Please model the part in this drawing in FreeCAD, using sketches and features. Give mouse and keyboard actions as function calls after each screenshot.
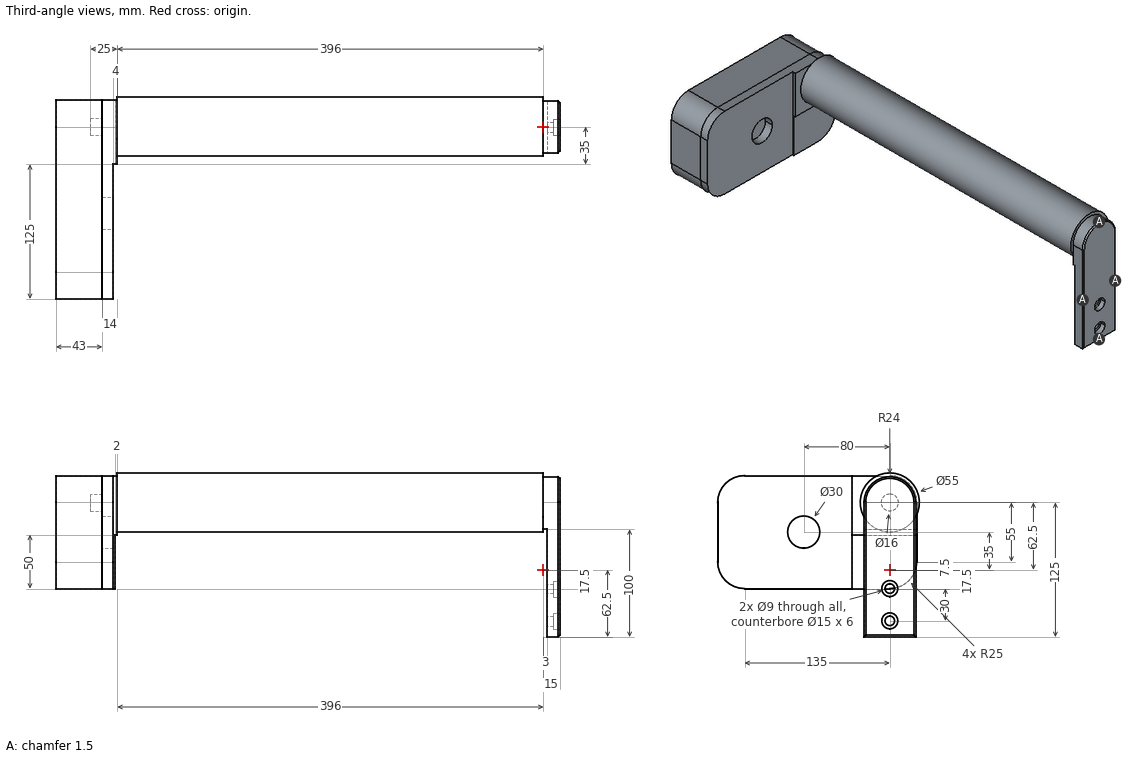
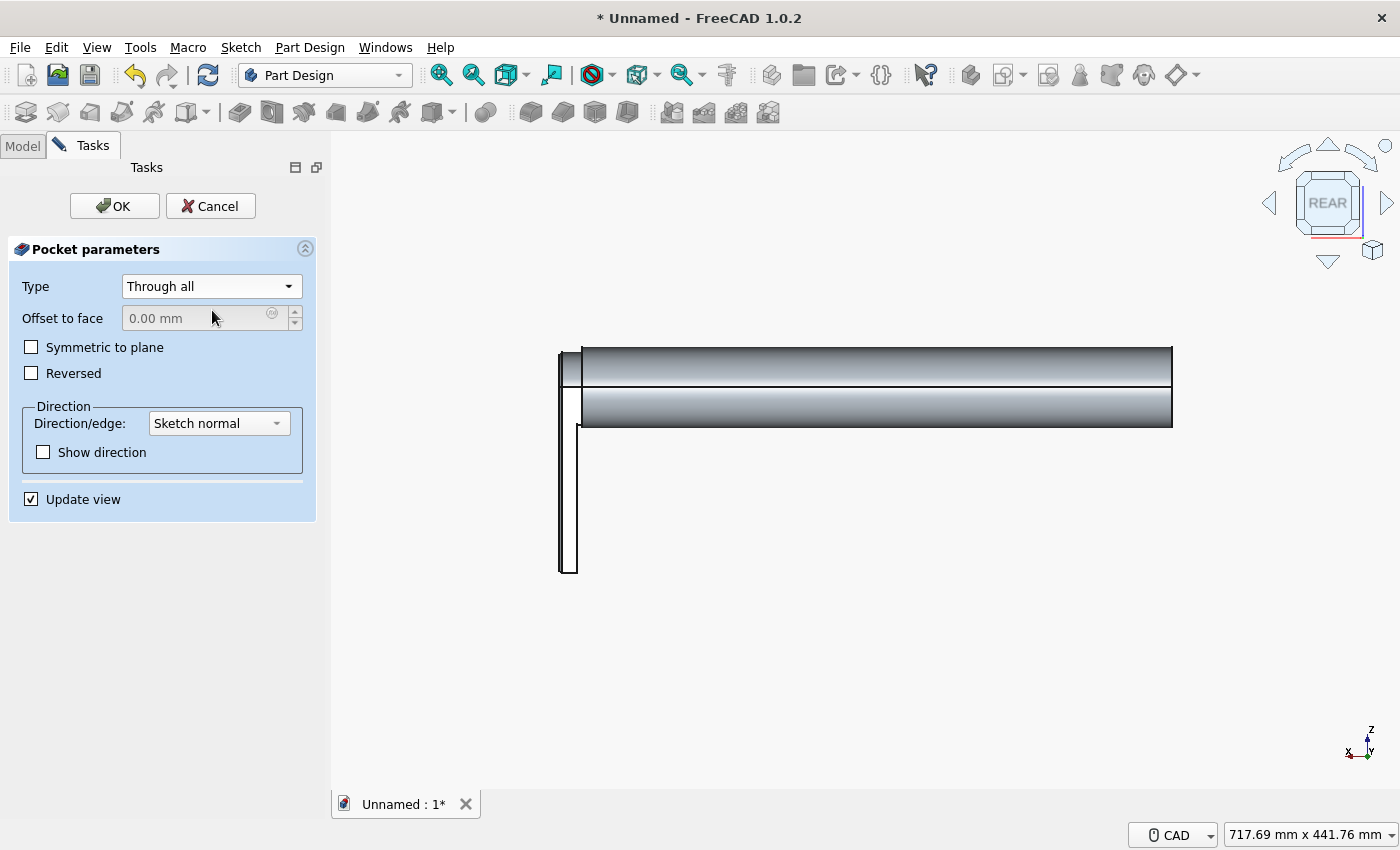
click(115, 206)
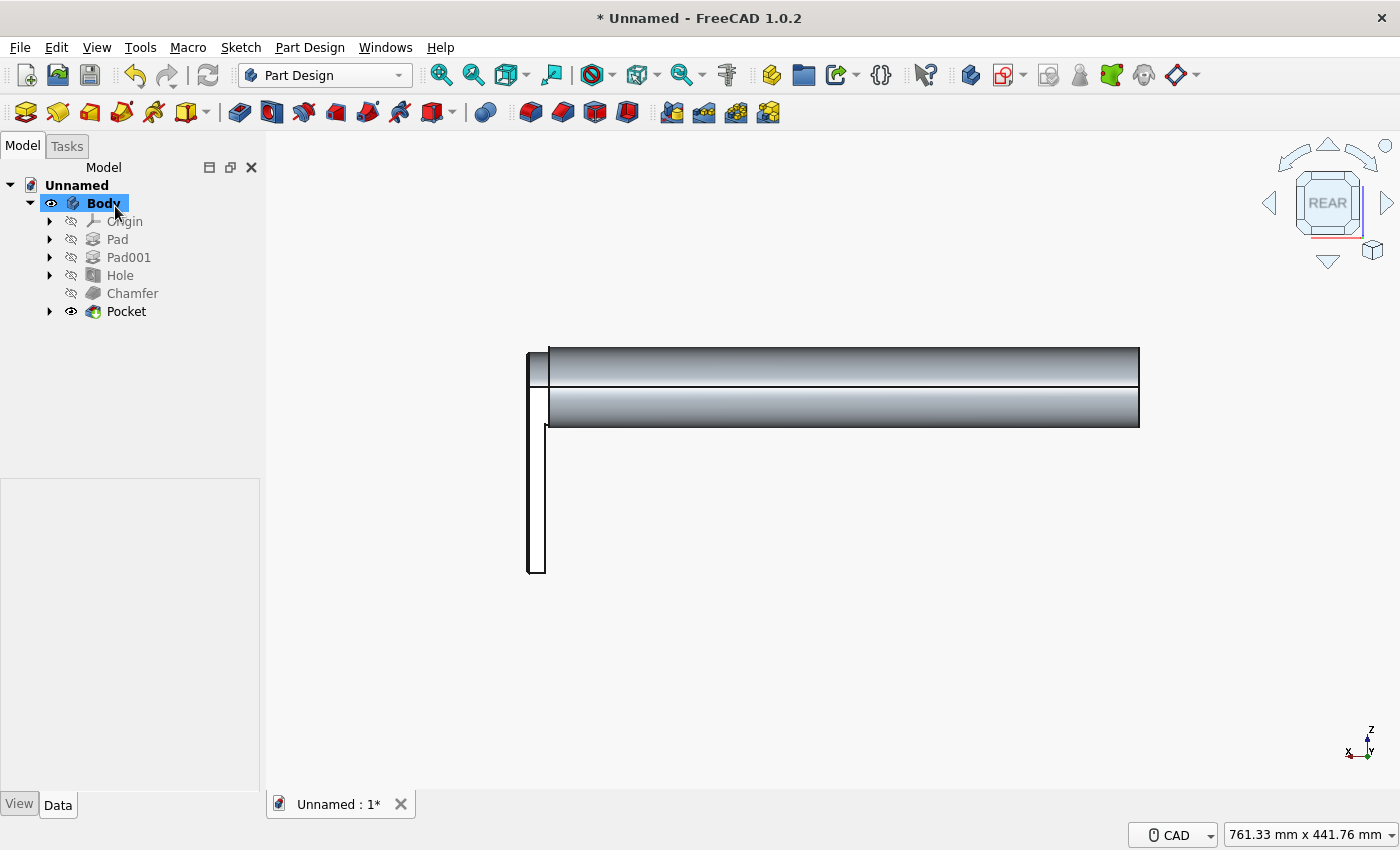
key(6)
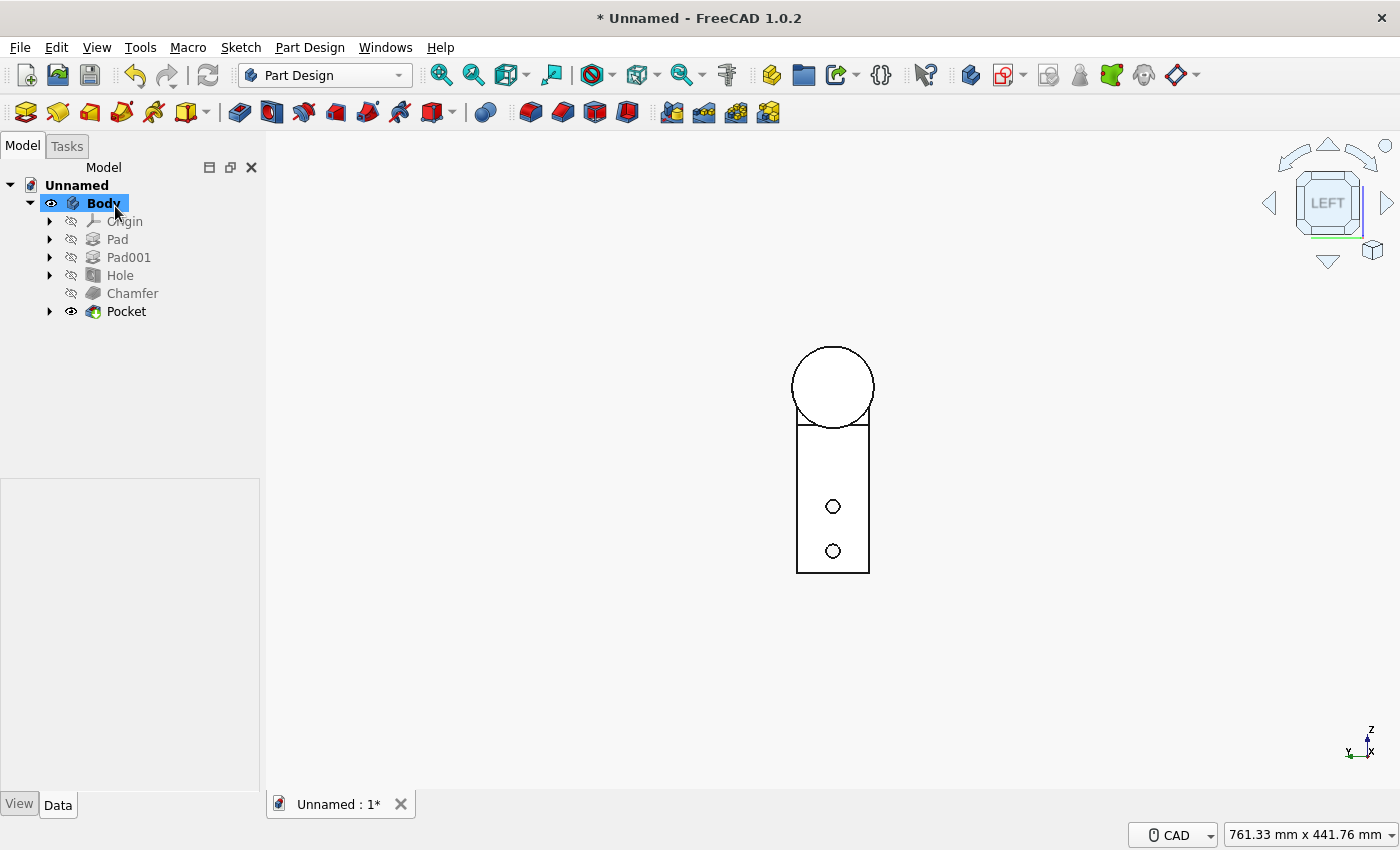
key(v)
key(f)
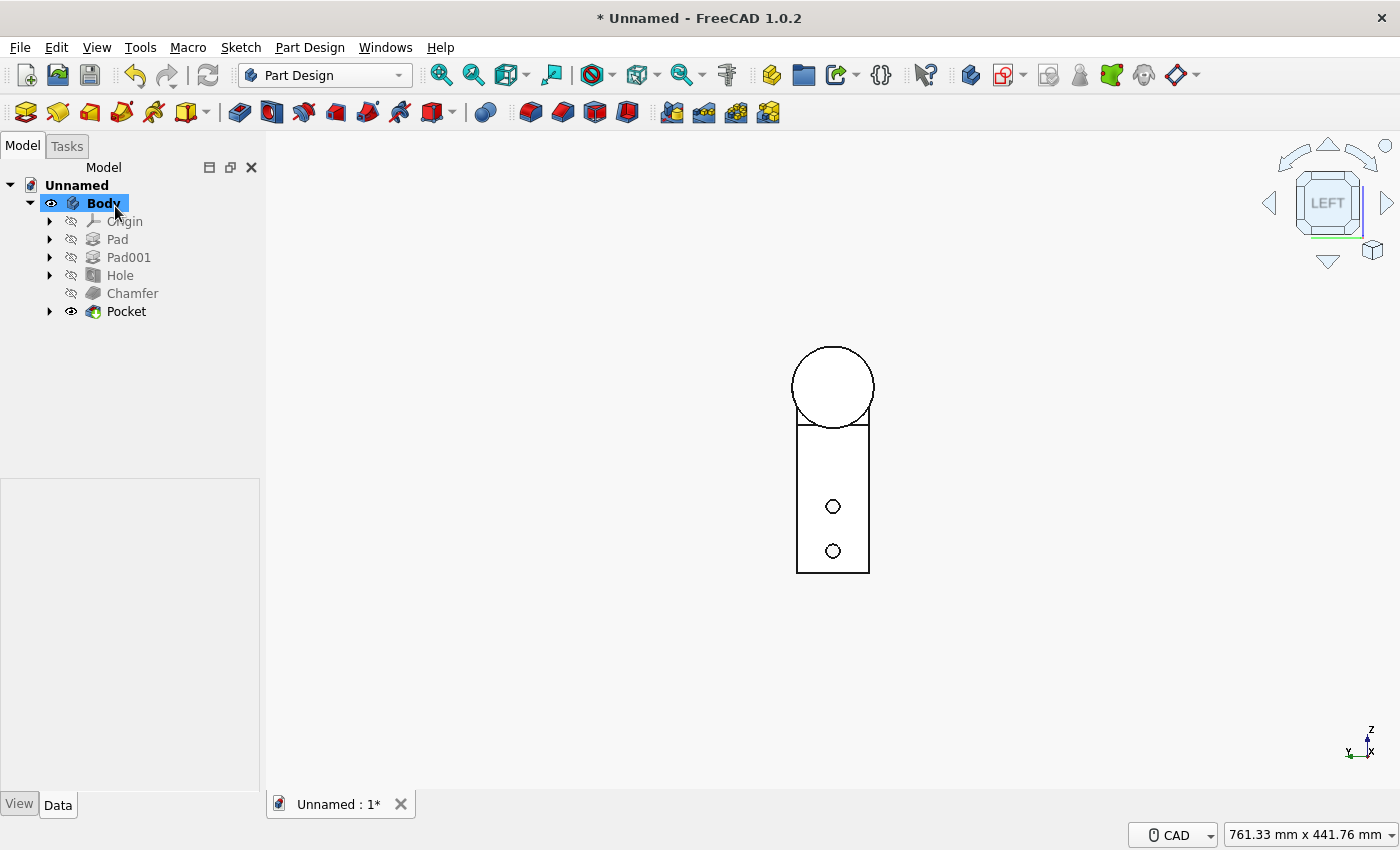
click(833, 386)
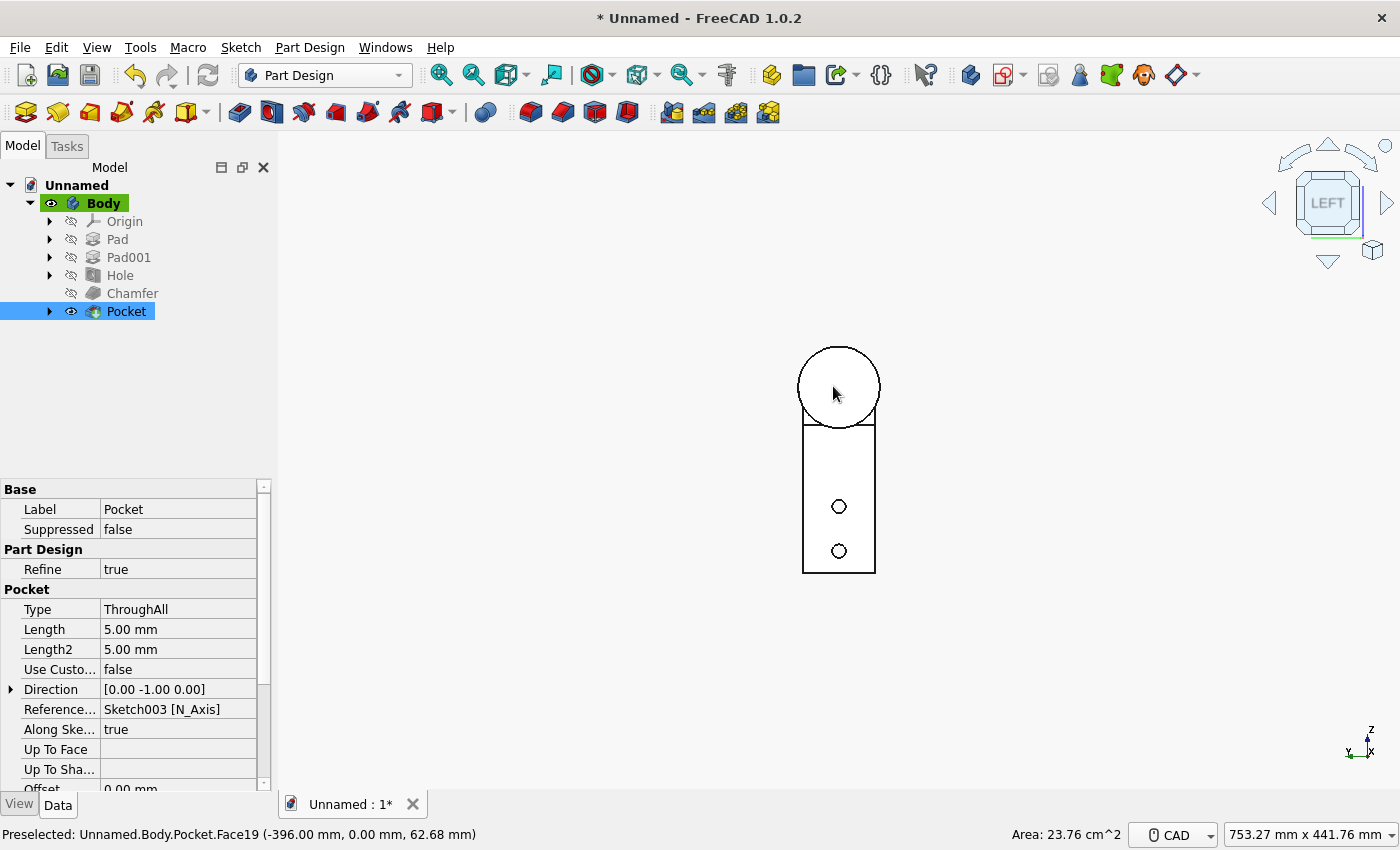
click(1004, 76)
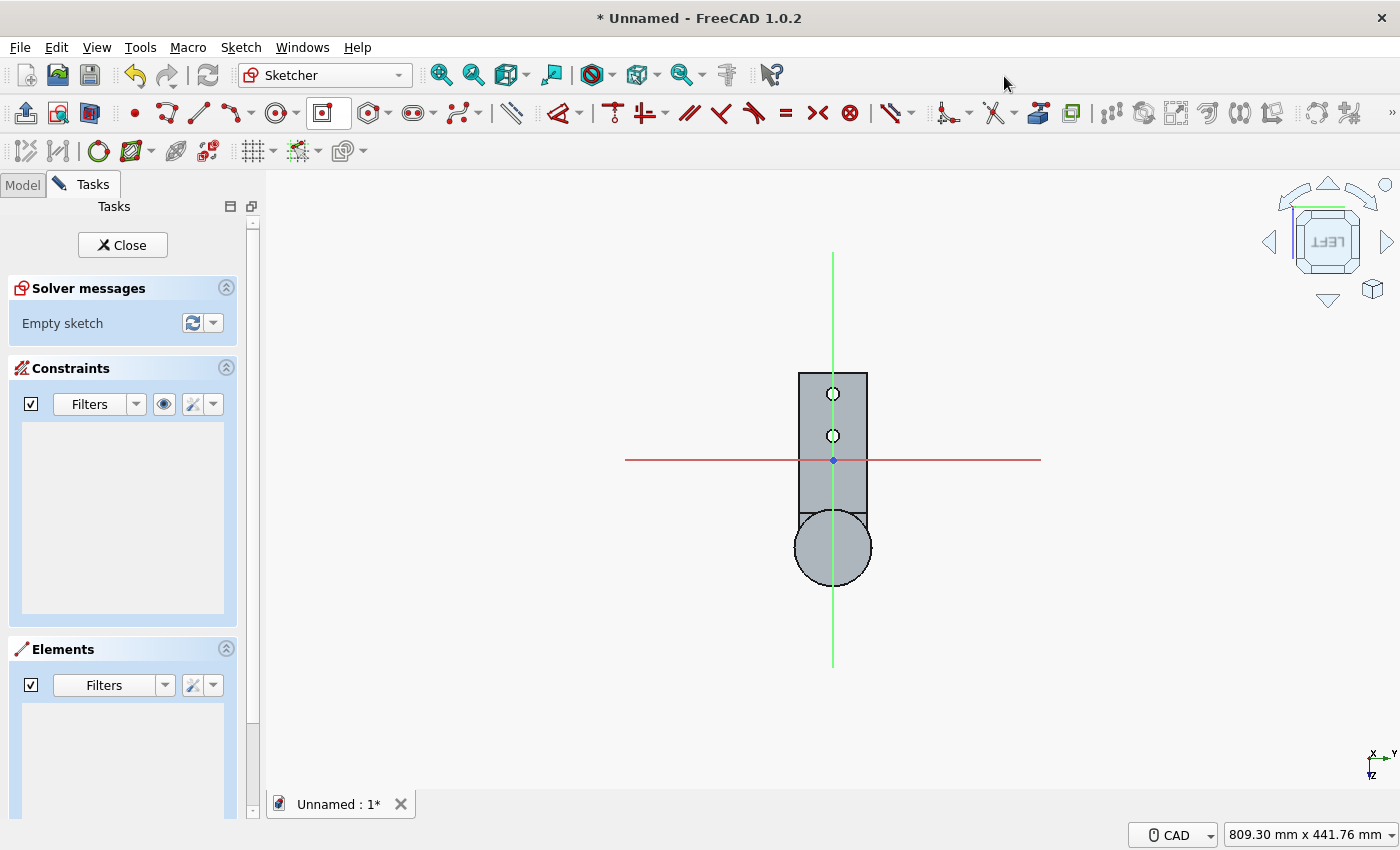
scroll(837, 552, up, 14)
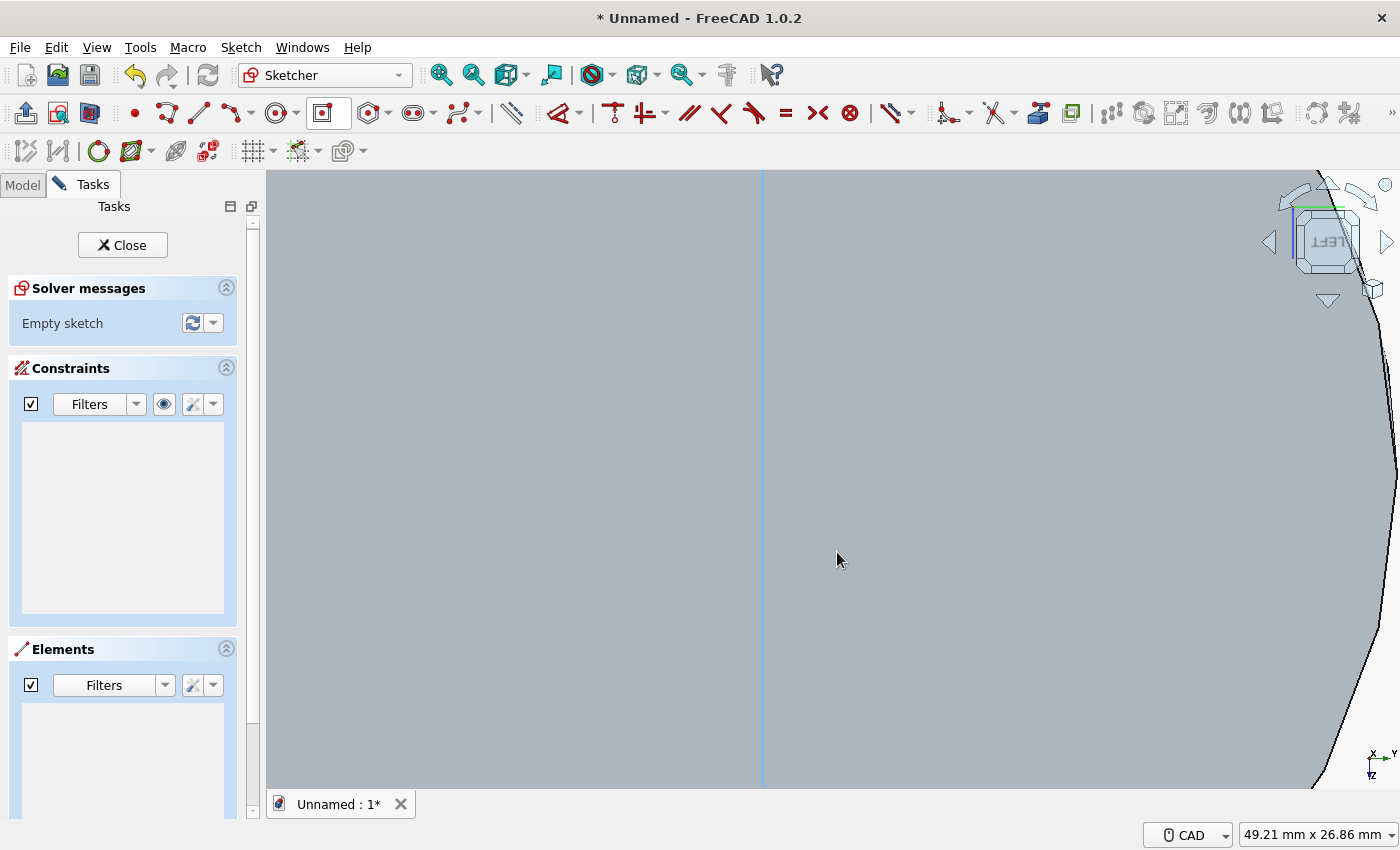
click(276, 114)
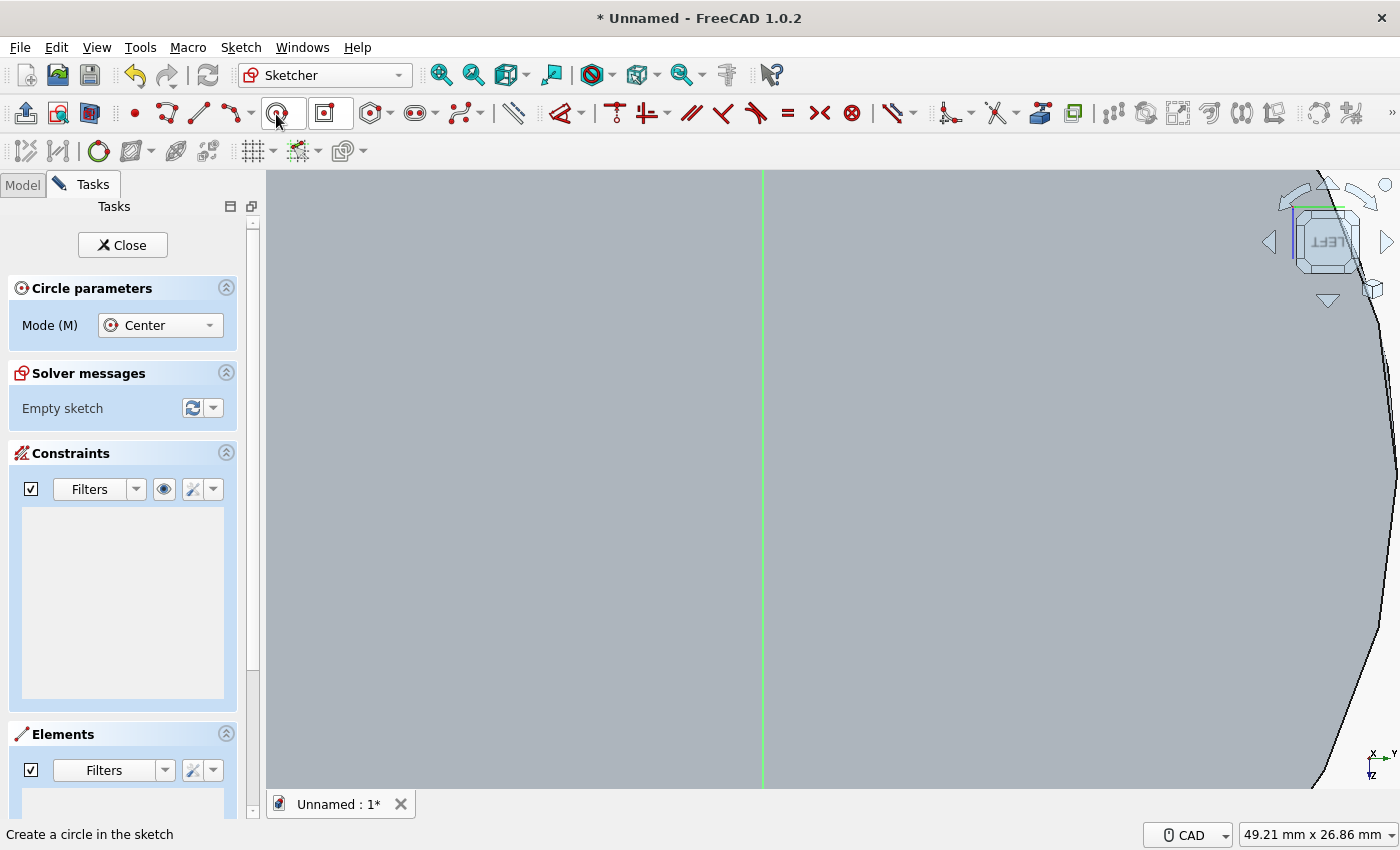
click(763, 475)
move(894, 345)